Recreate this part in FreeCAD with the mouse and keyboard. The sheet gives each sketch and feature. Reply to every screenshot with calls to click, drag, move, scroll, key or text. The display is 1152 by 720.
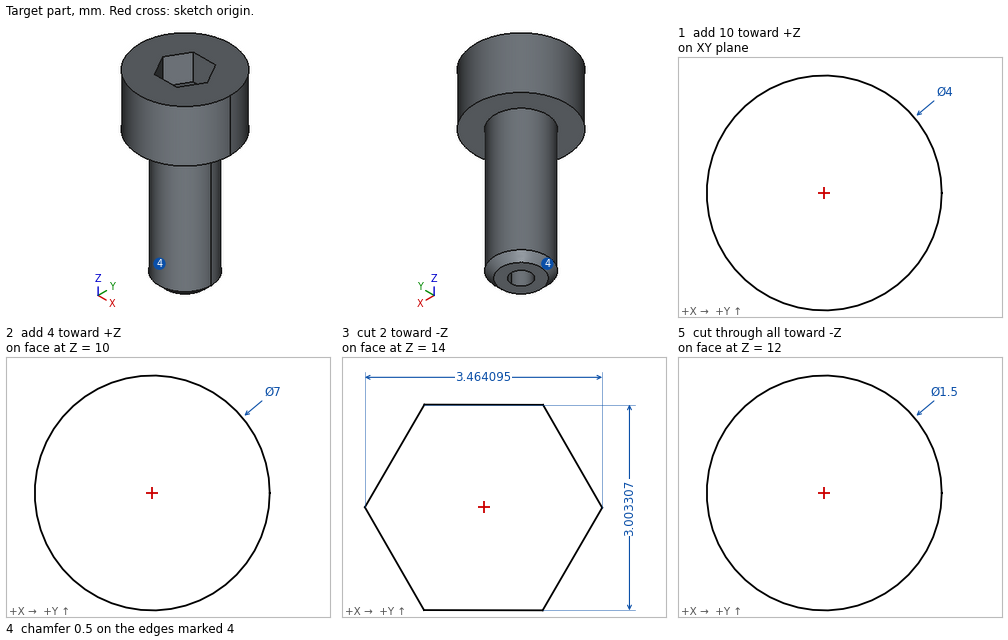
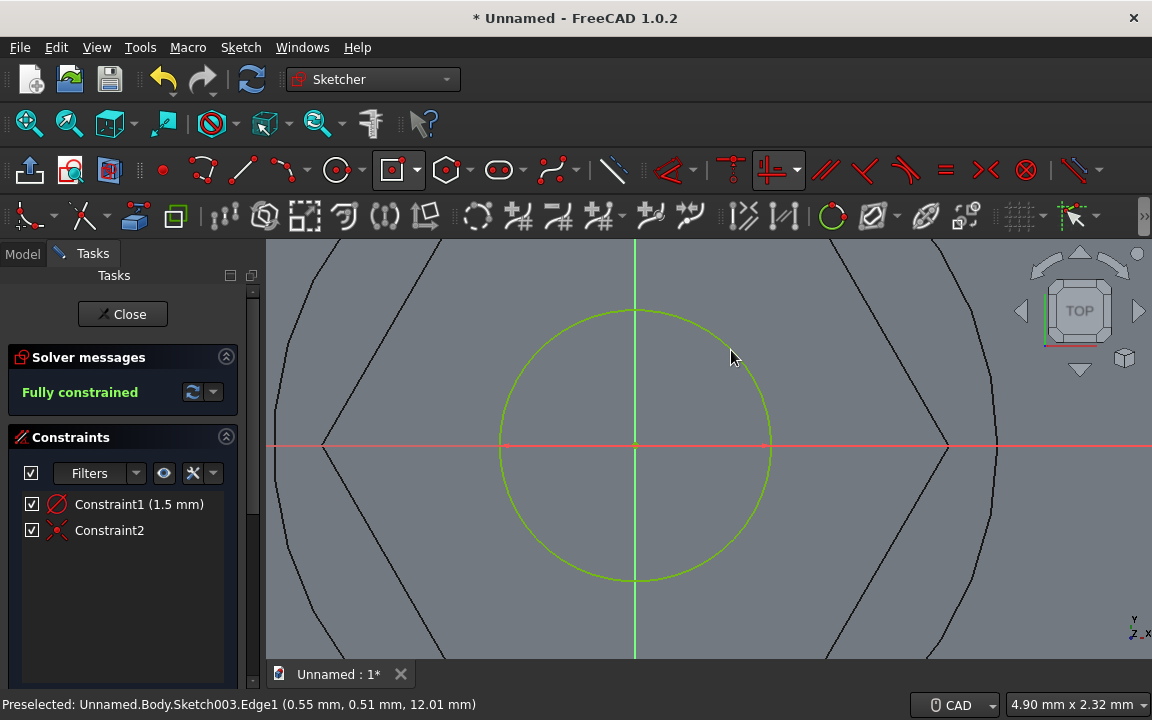
click(123, 314)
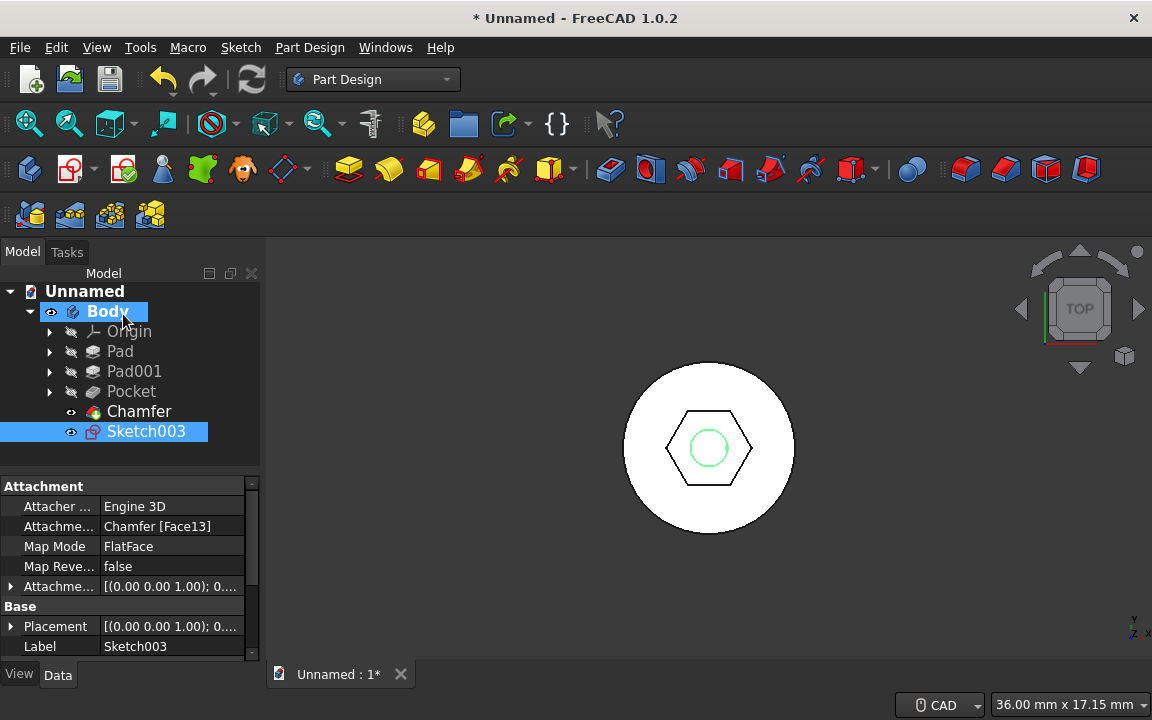
click(612, 170)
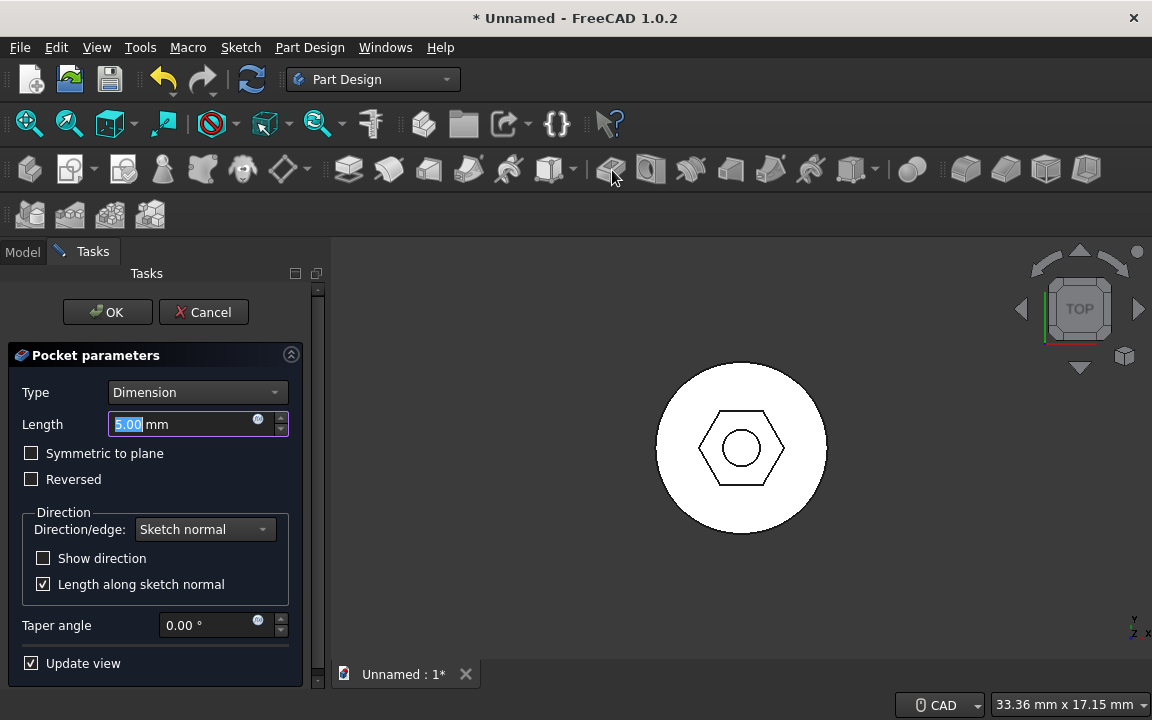
click(198, 392)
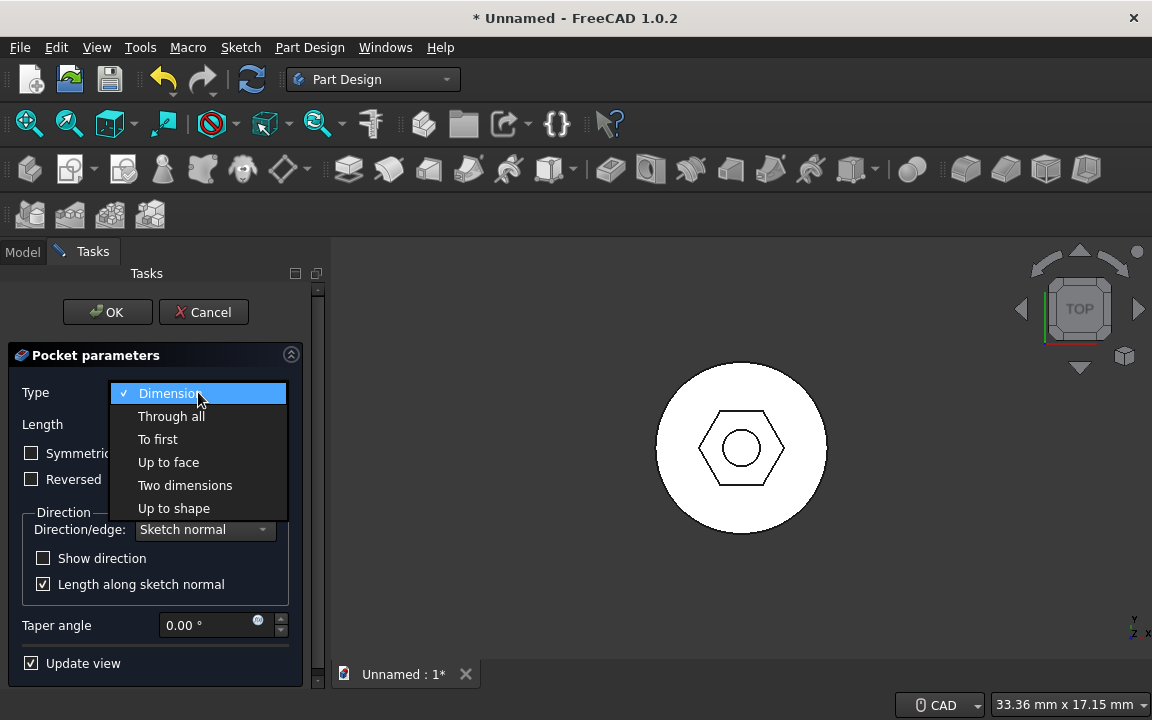
click(198, 416)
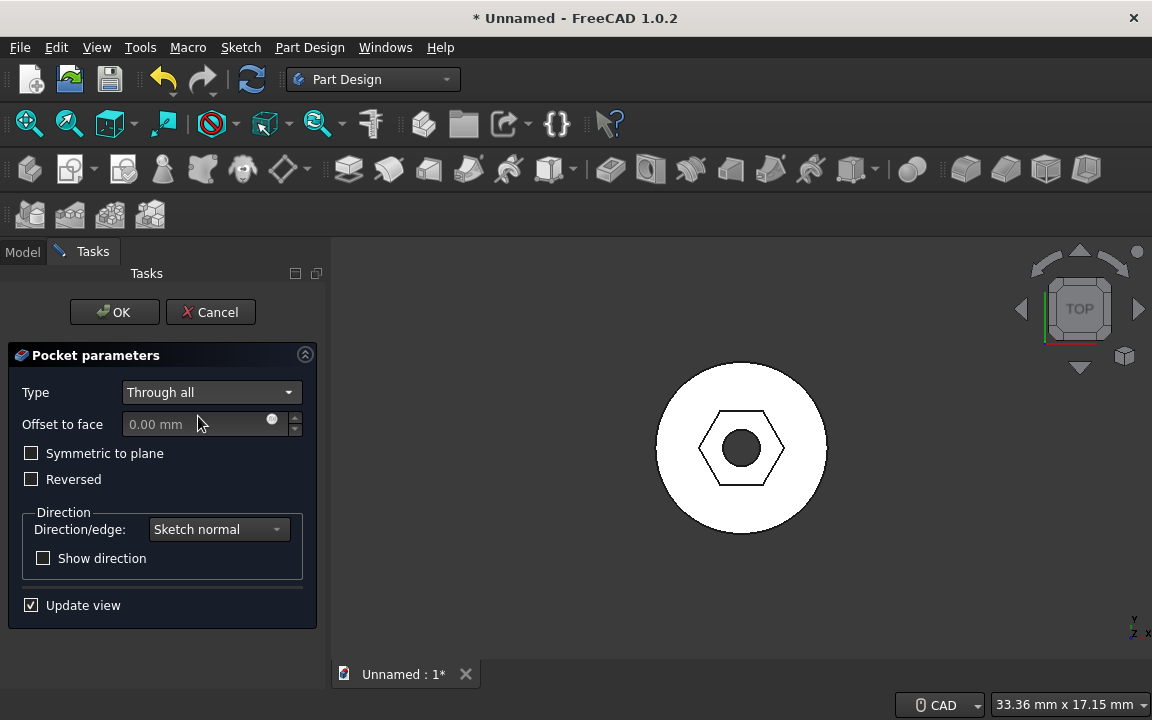
click(115, 312)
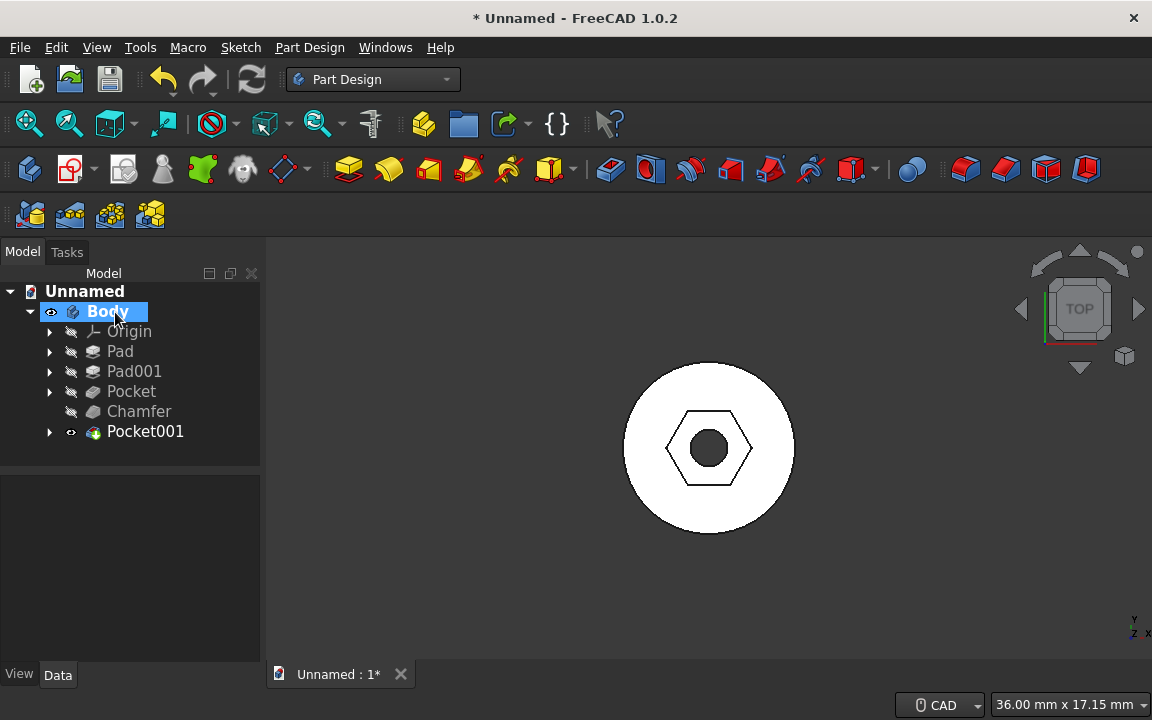
key(0)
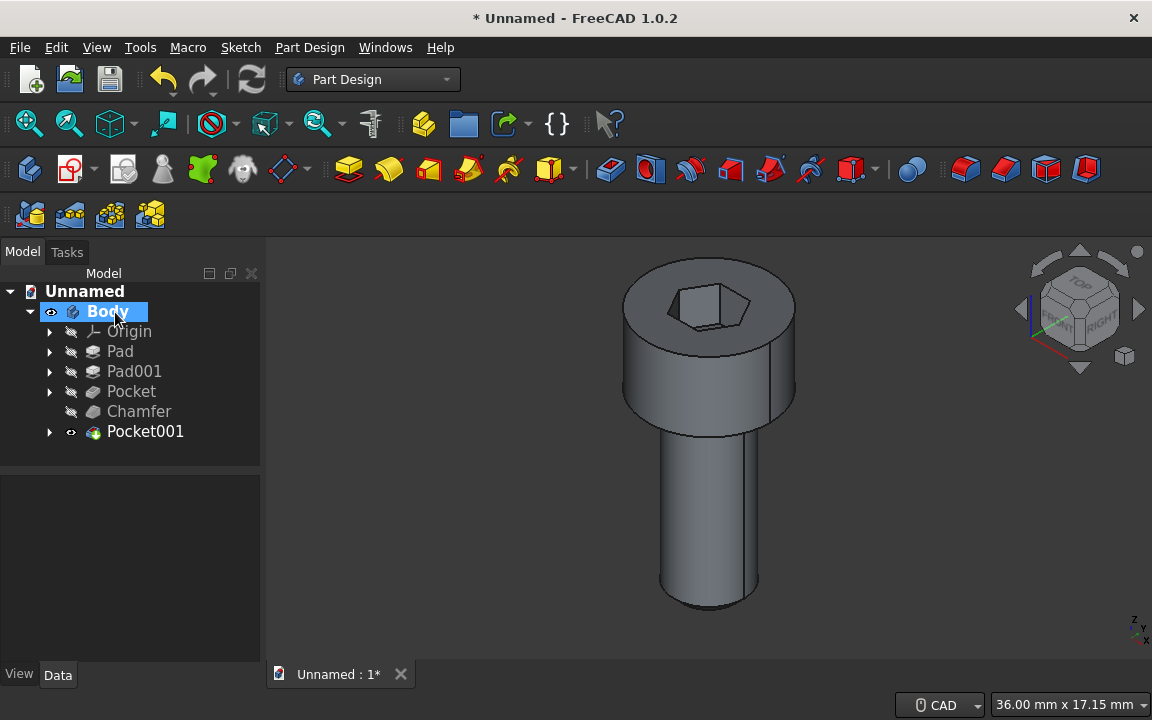
key(v)
key(f)